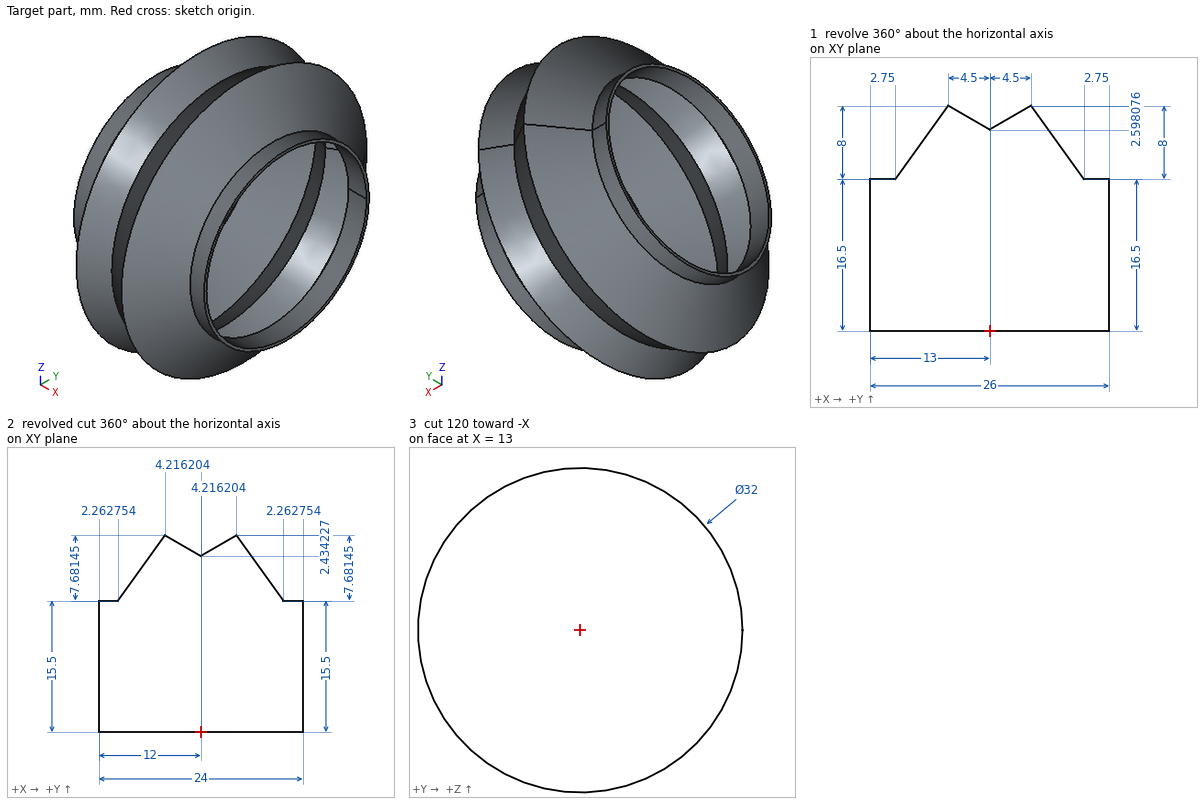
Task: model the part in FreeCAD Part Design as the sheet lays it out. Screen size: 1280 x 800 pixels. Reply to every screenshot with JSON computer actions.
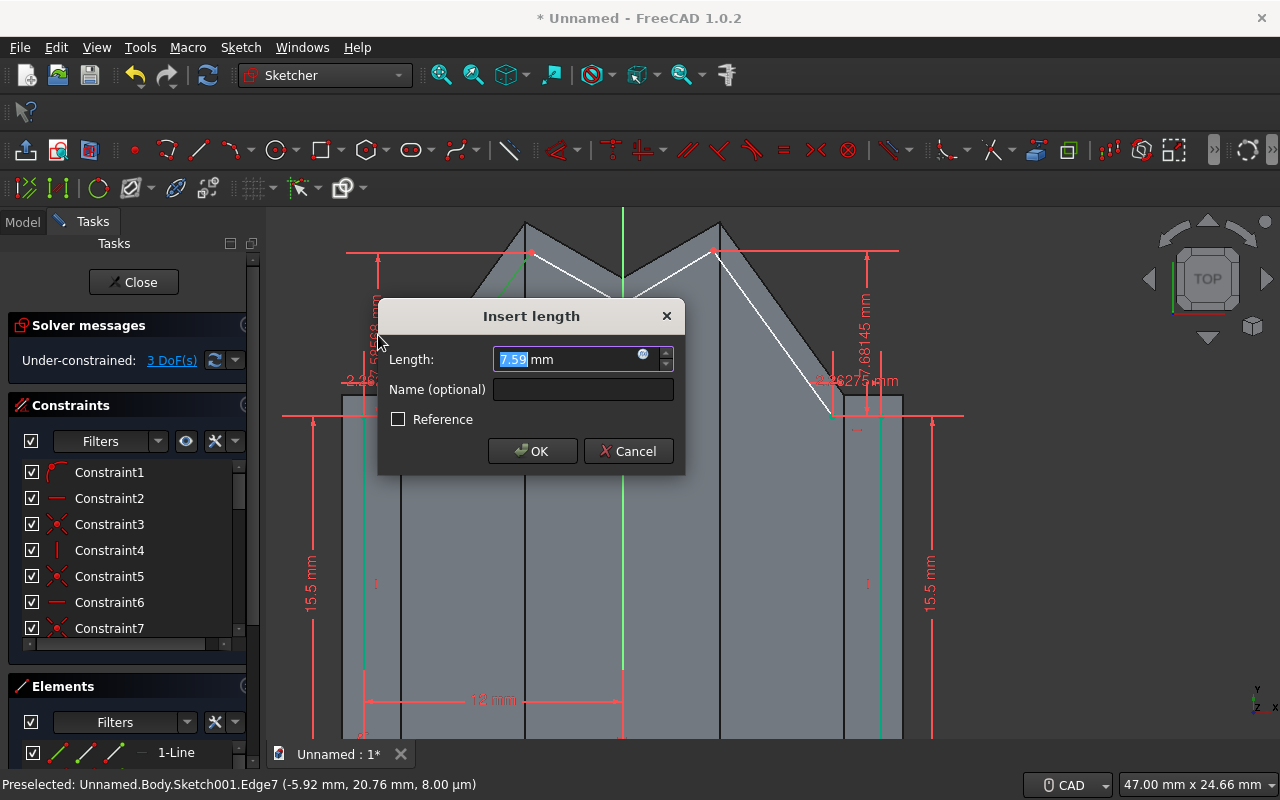
{"action": "type", "text": "7.68145"}
{"action": "key", "text": "Return"}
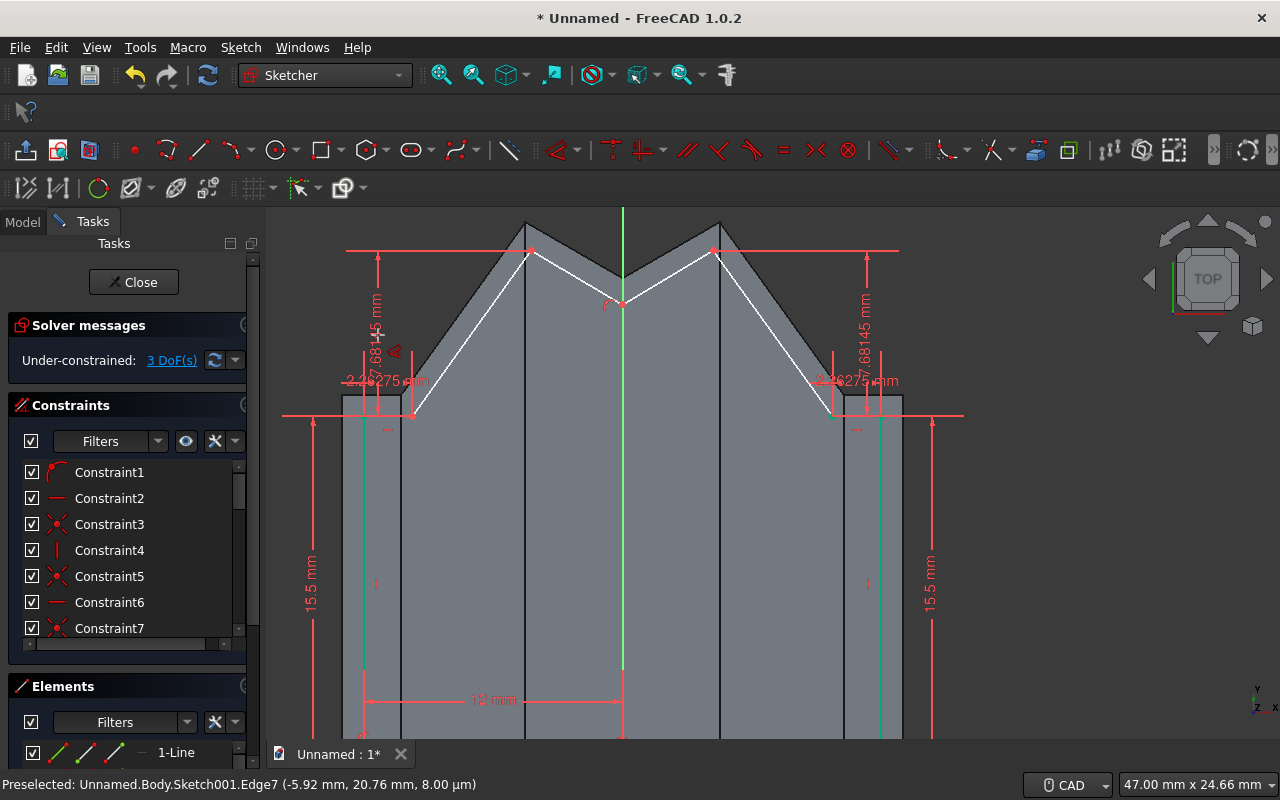
{"action": "left_click", "coordinate": [713, 251]}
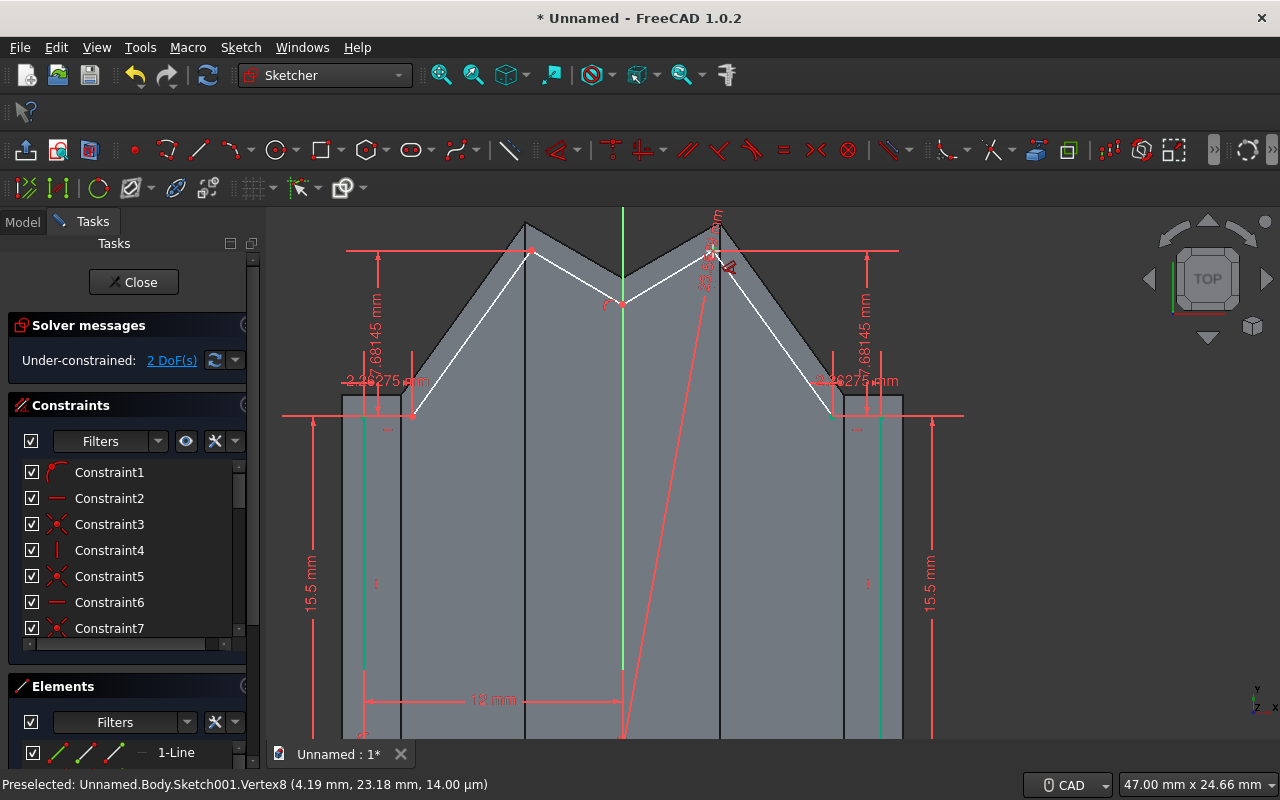
{"action": "key", "text": "Escape"}
{"action": "key", "text": "Escape"}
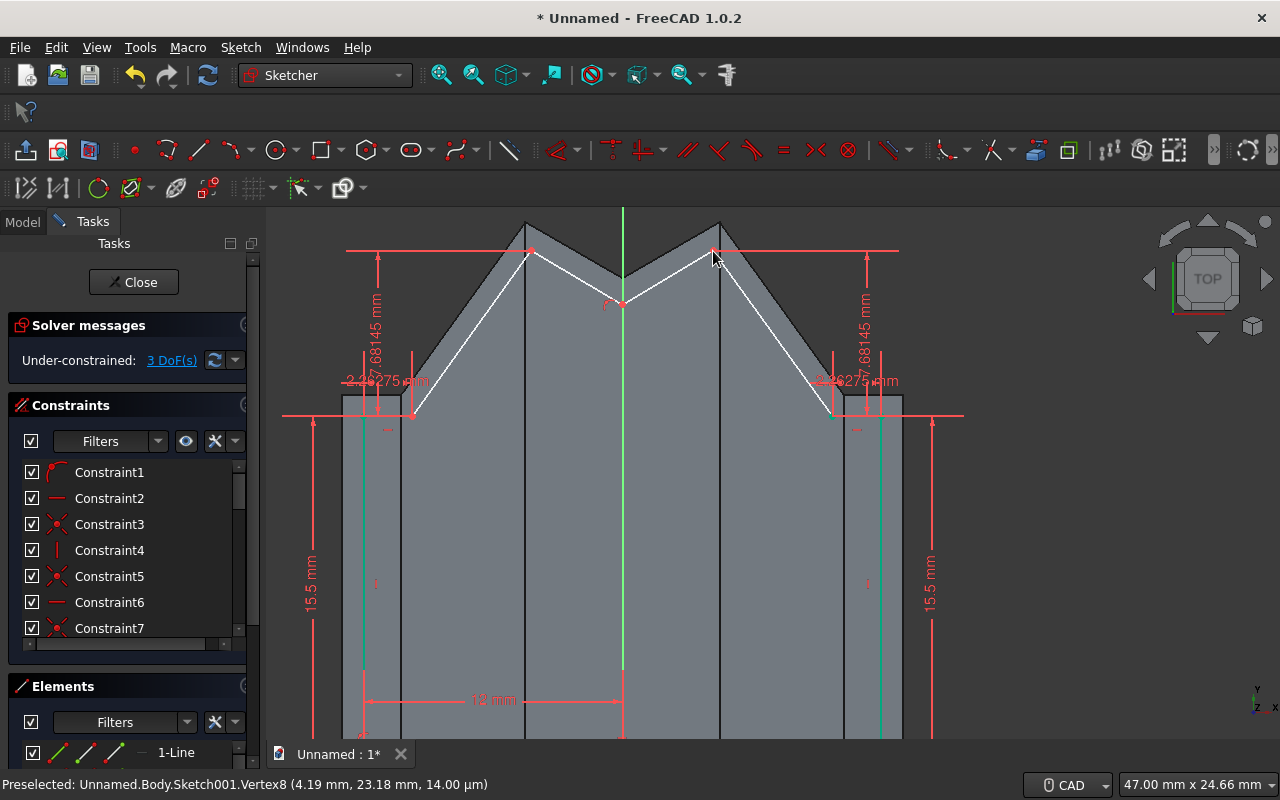
{"action": "left_click", "coordinate": [713, 251]}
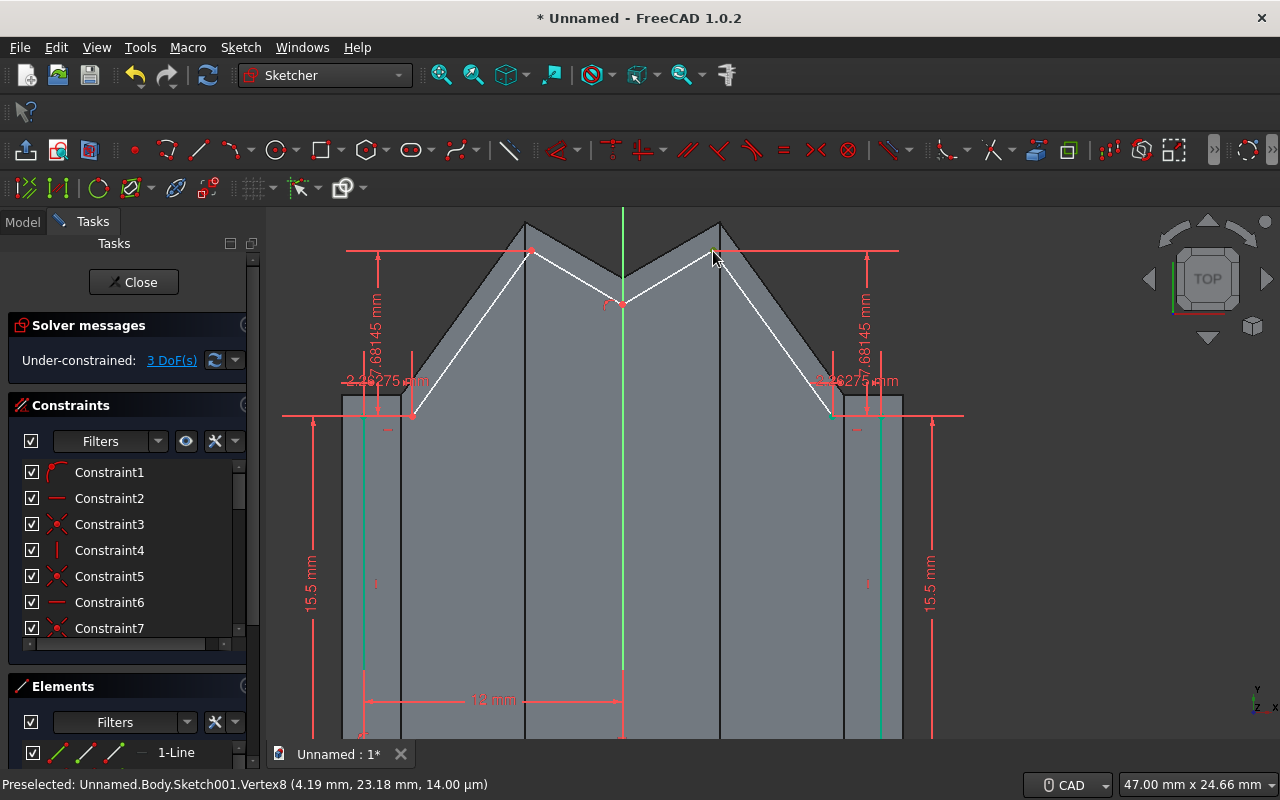
{"action": "key", "text": "l"}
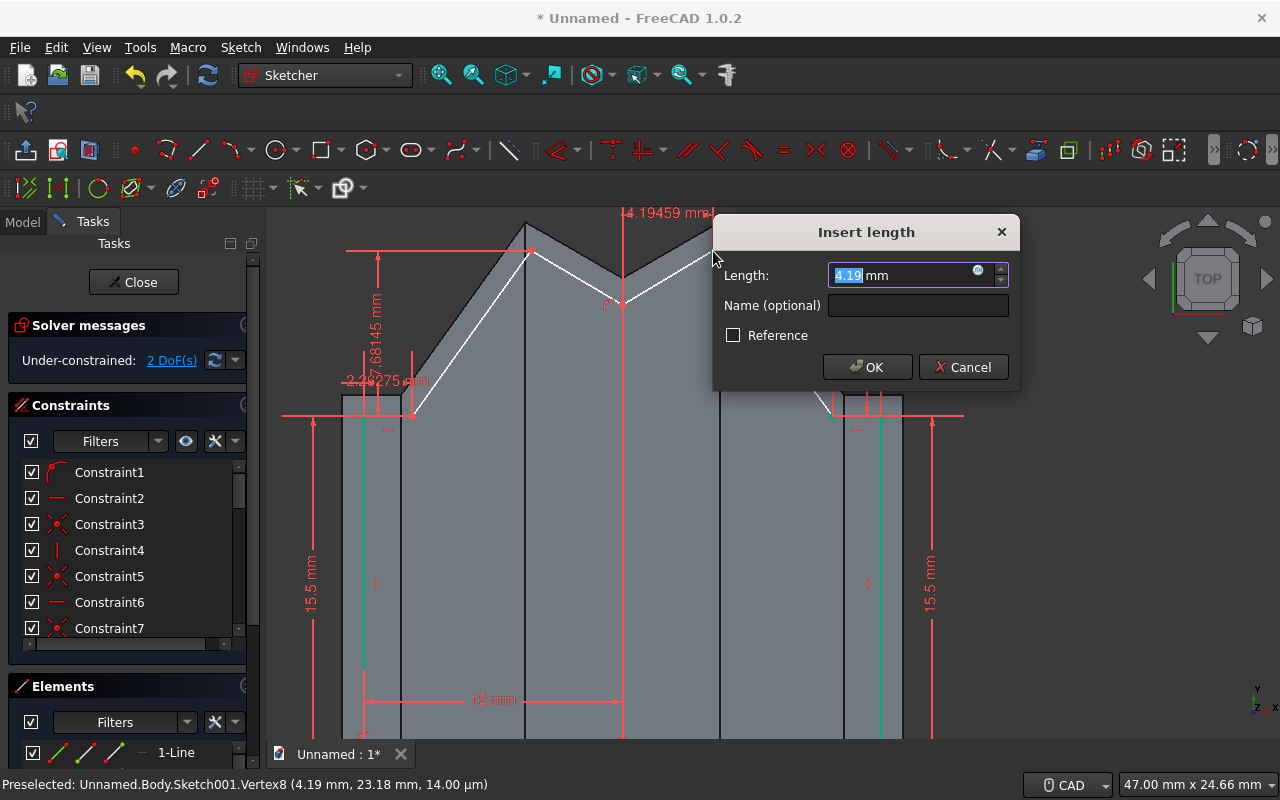
{"action": "type", "text": "4.216204"}
{"action": "key", "text": "Return"}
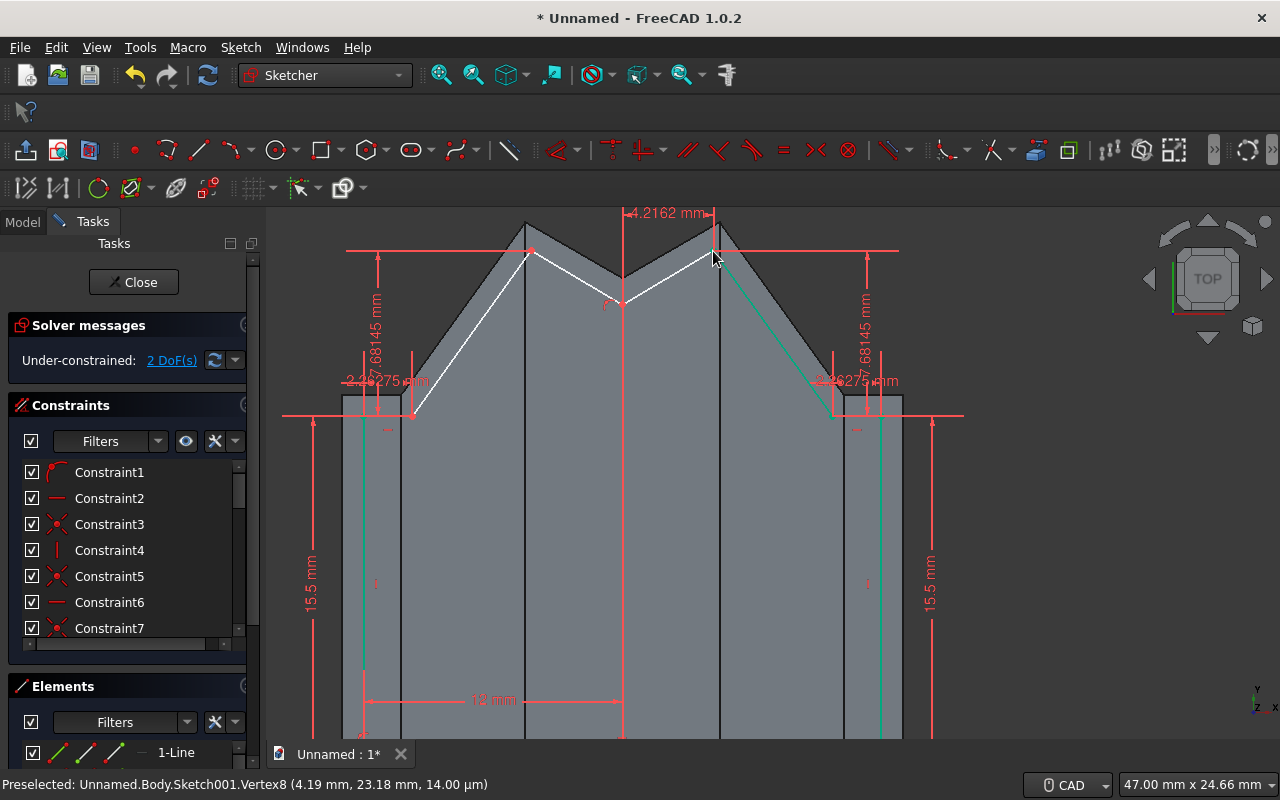
{"action": "left_click", "coordinate": [531, 251]}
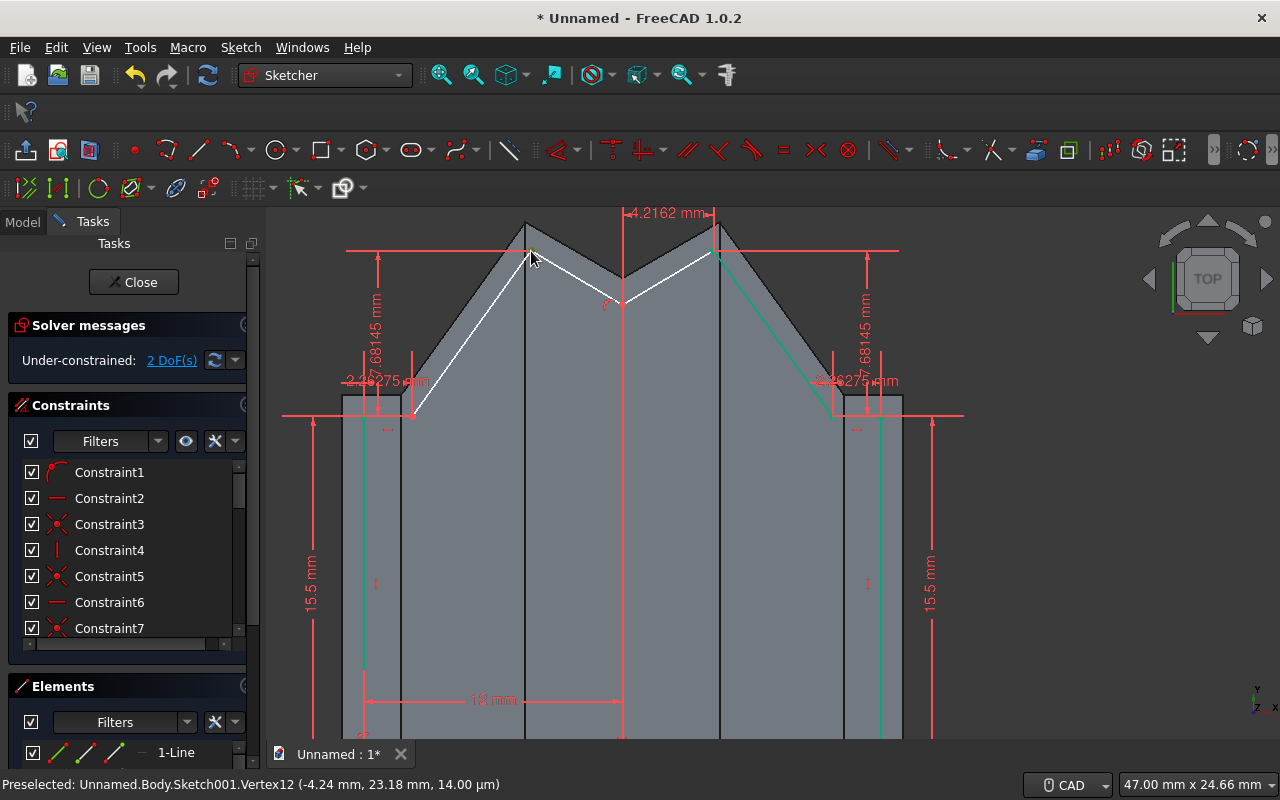
{"action": "left_click", "coordinate": [580, 150]}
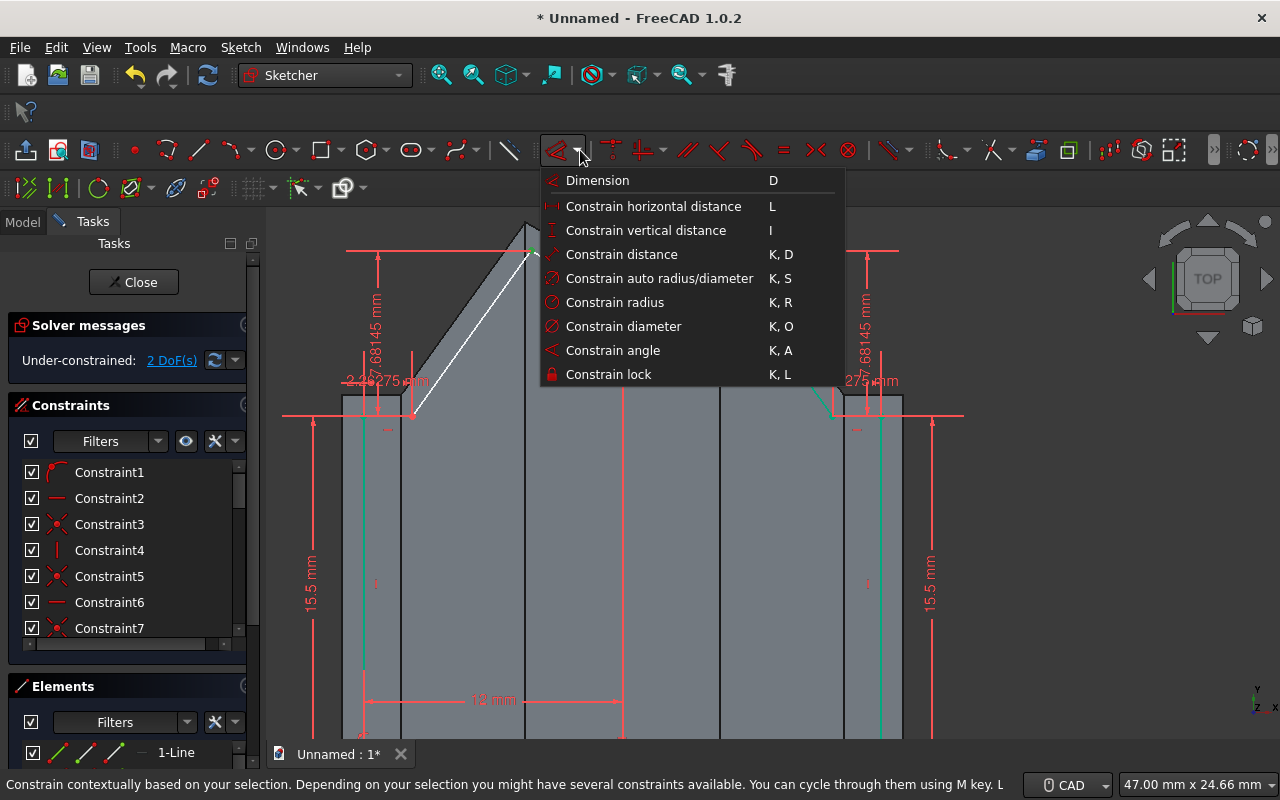
{"action": "left_click", "coordinate": [693, 206]}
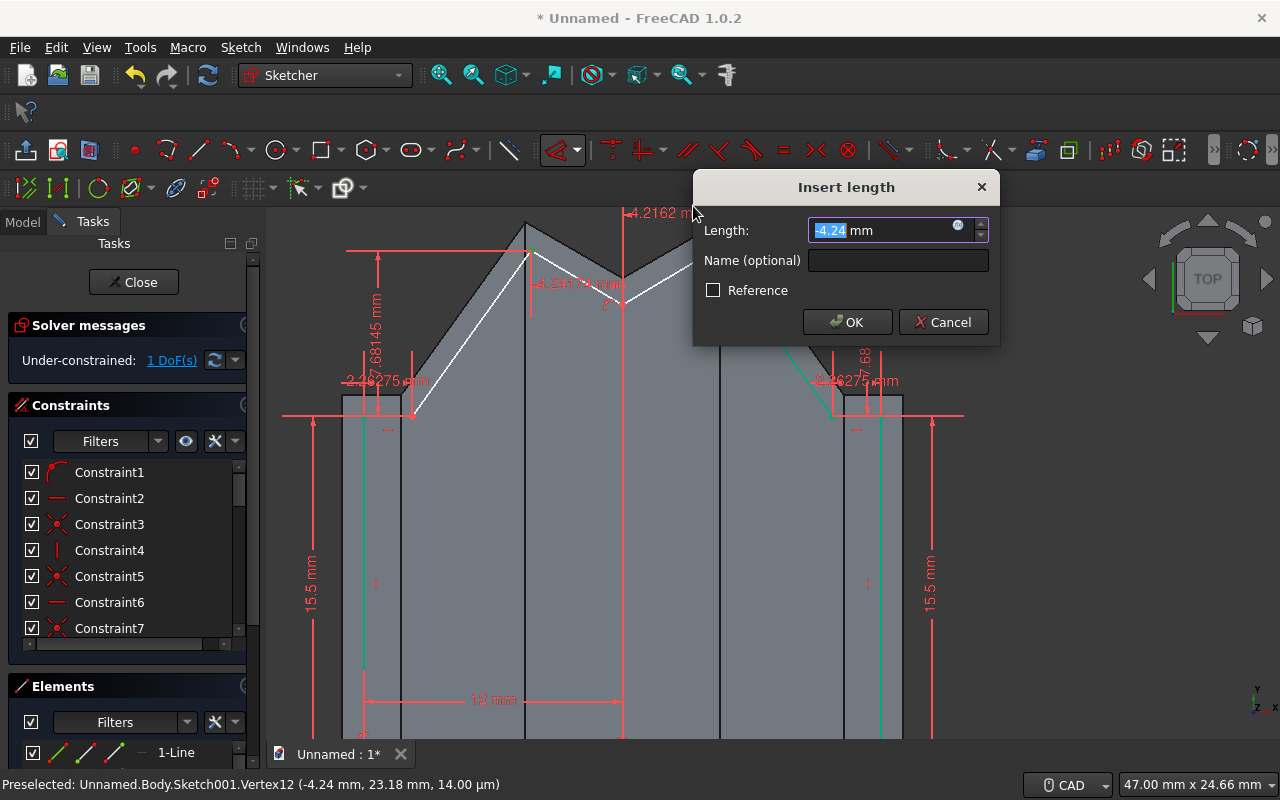
{"action": "type", "text": "-4.216204"}
{"action": "key", "text": "Return"}